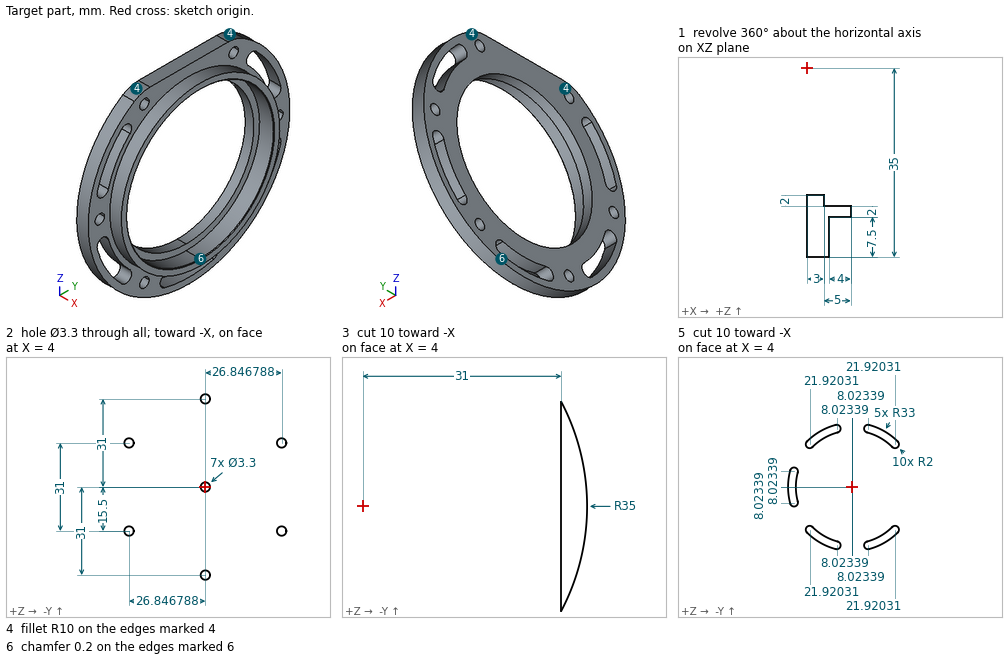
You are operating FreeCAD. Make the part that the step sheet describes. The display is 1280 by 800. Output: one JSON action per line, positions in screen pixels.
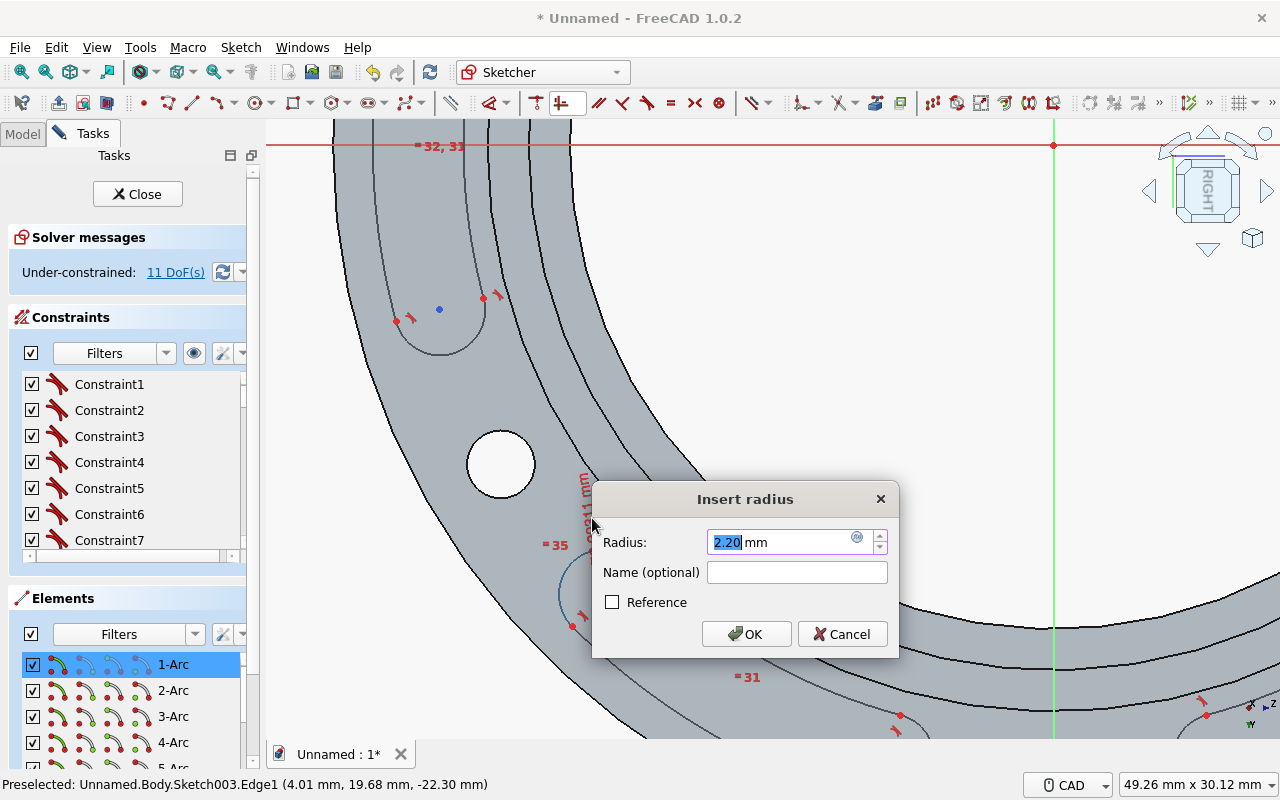
{"action": "type", "text": "2"}
{"action": "key", "text": "Return"}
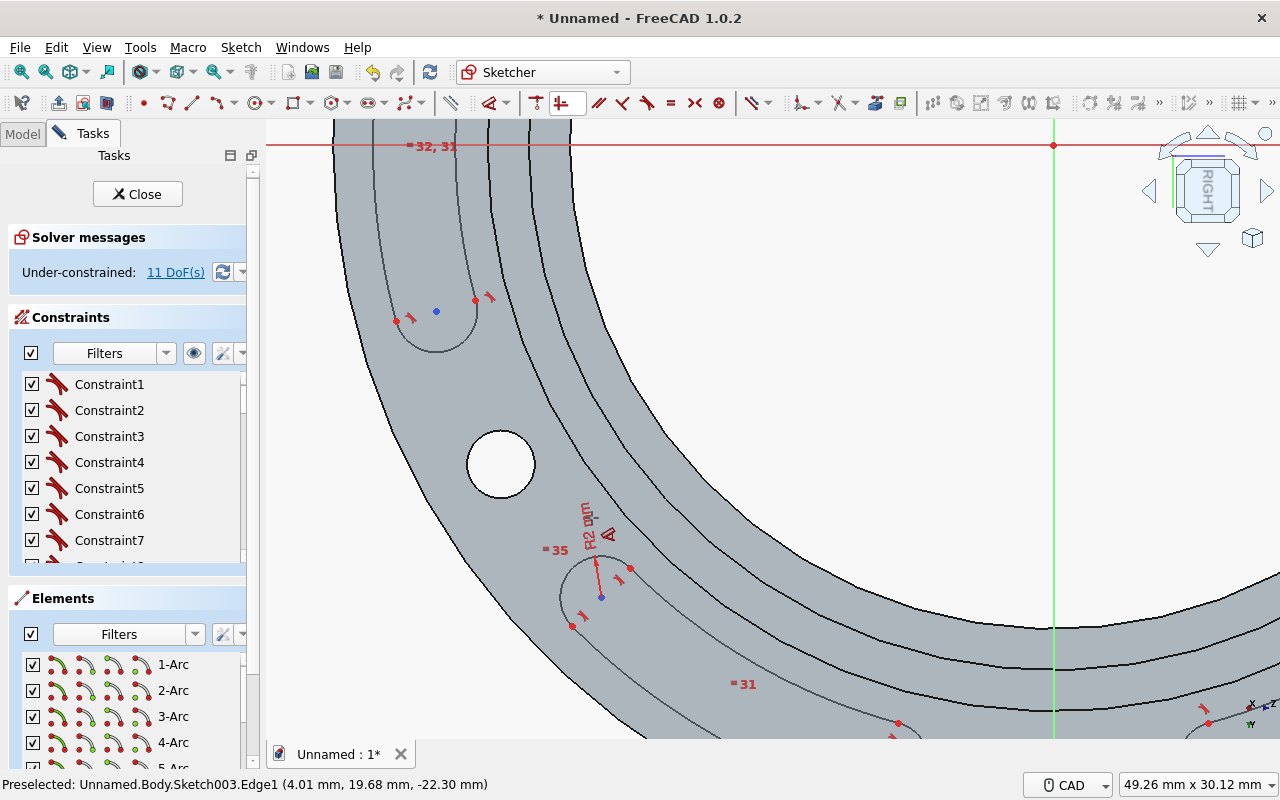
{"action": "left_click", "coordinate": [654, 696]}
{"action": "left_click", "coordinate": [410, 451]}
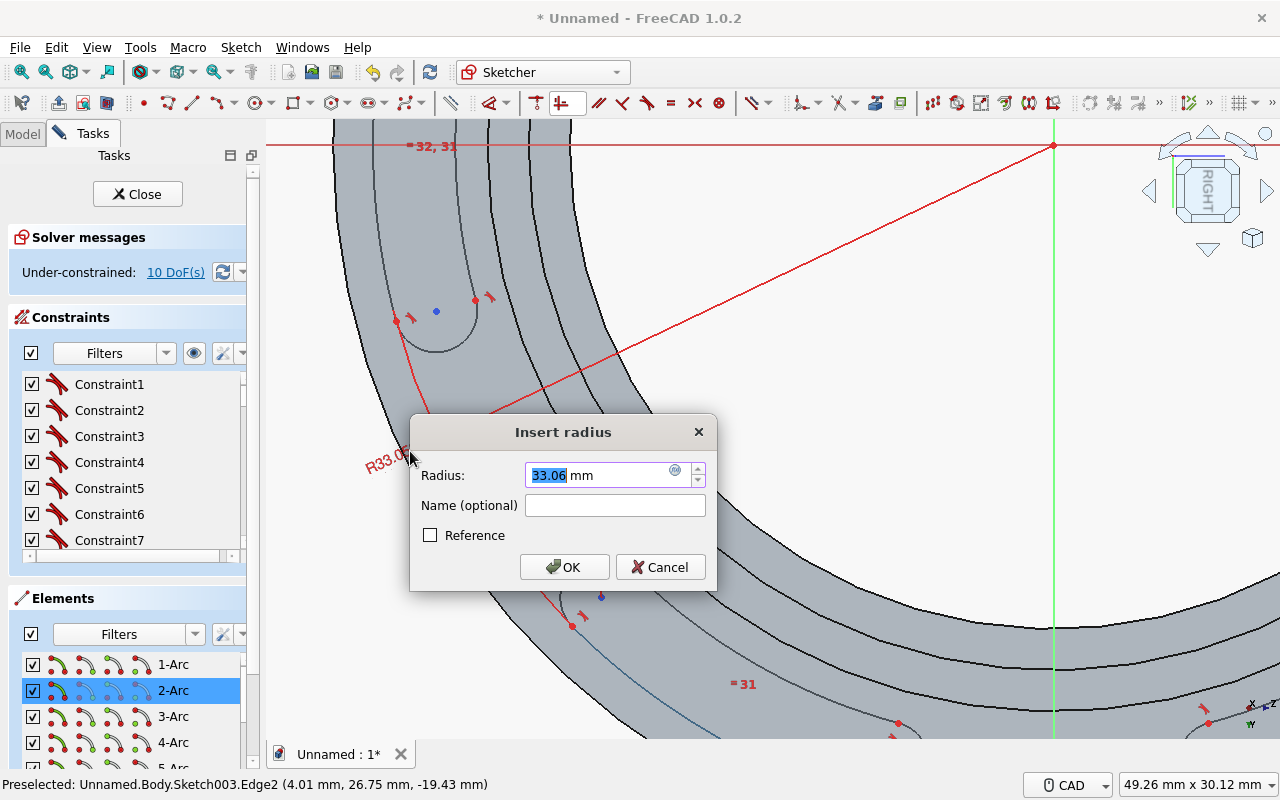
{"action": "type", "text": "33"}
{"action": "key", "text": "Return"}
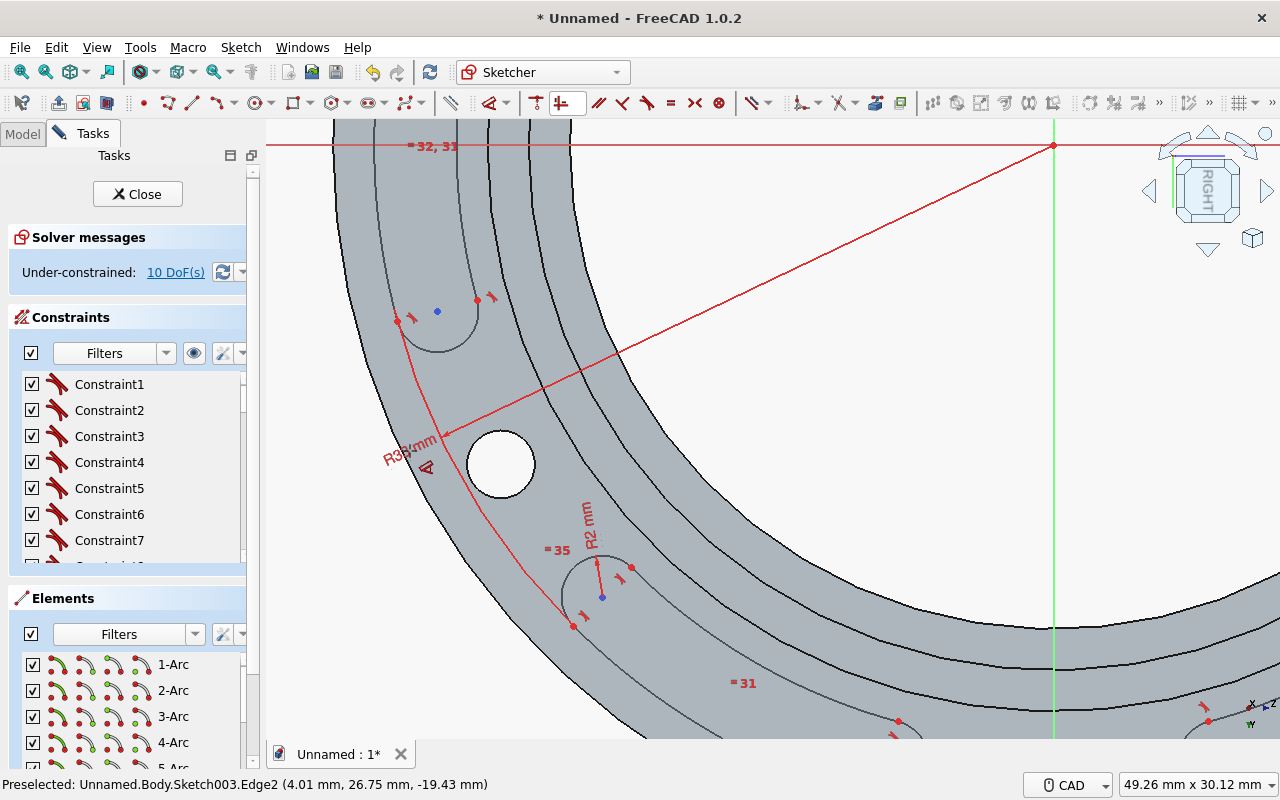
{"action": "scroll", "coordinate": [597, 551], "scroll_direction": "down", "scroll_amount": 6}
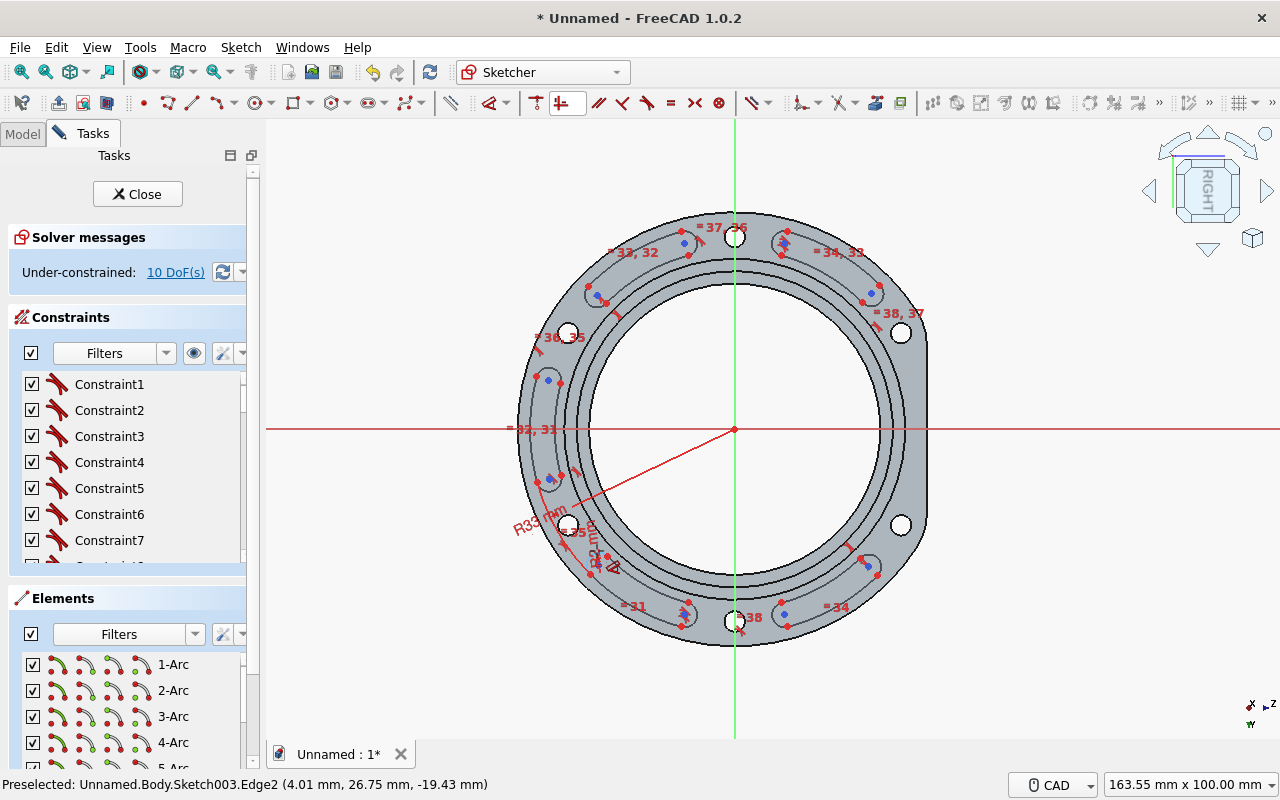
{"action": "left_click", "coordinate": [685, 615]}
{"action": "left_click", "coordinate": [710, 649]}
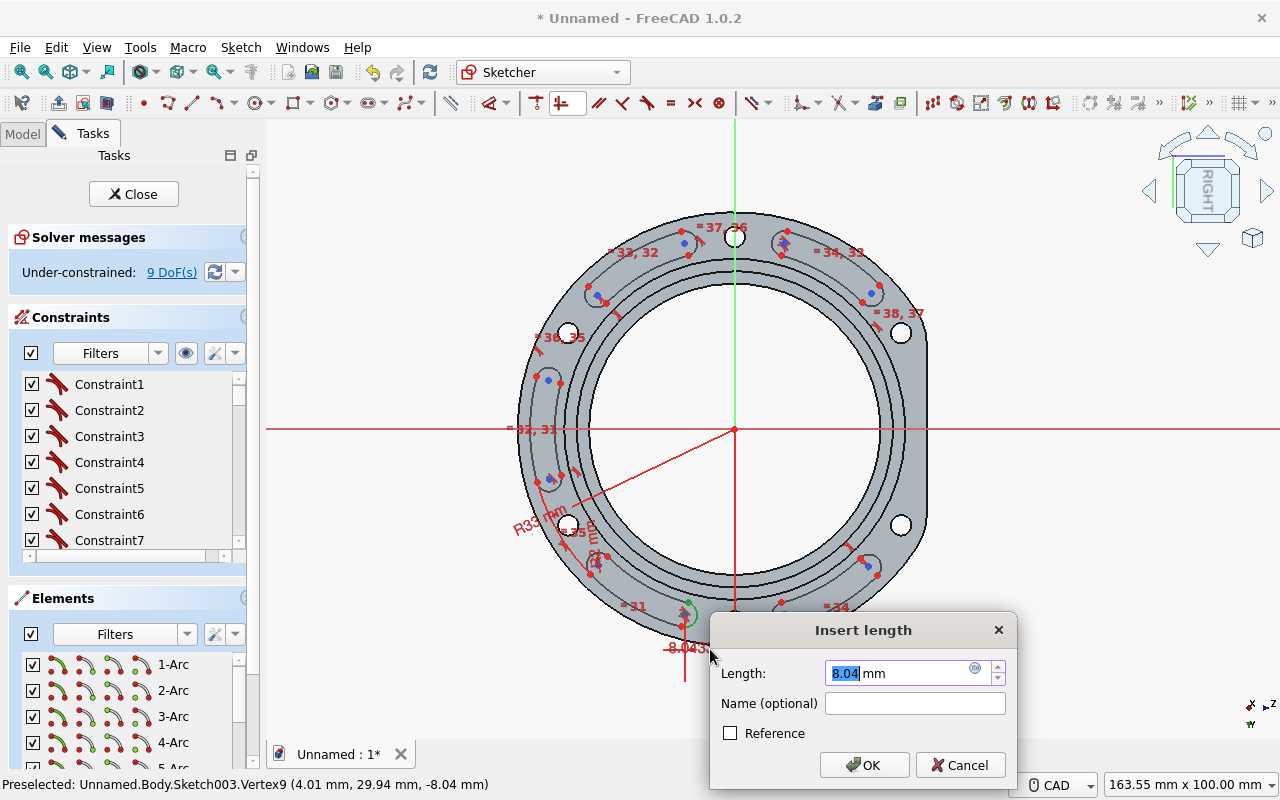
{"action": "type", "text": "8.02339"}
{"action": "key", "text": "Return"}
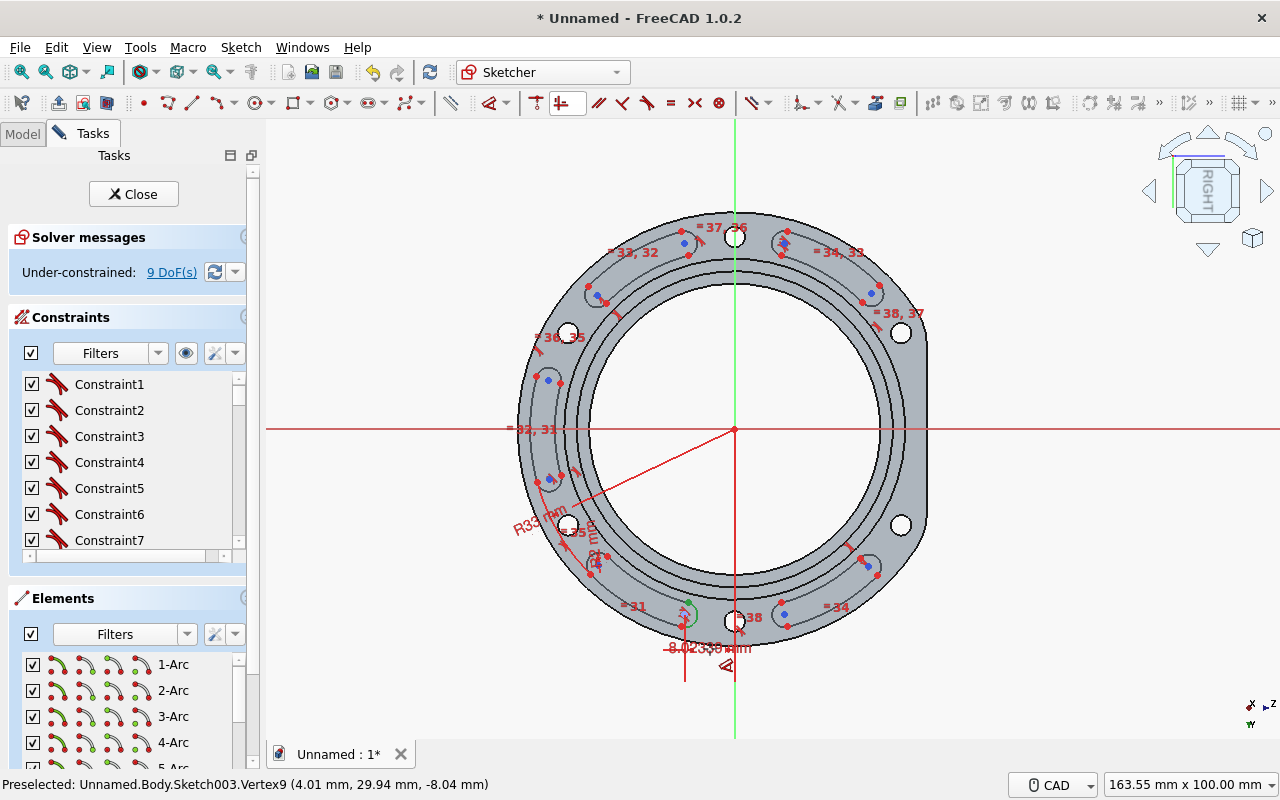
{"action": "left_click", "coordinate": [549, 380]}
{"action": "left_click", "coordinate": [515, 405]}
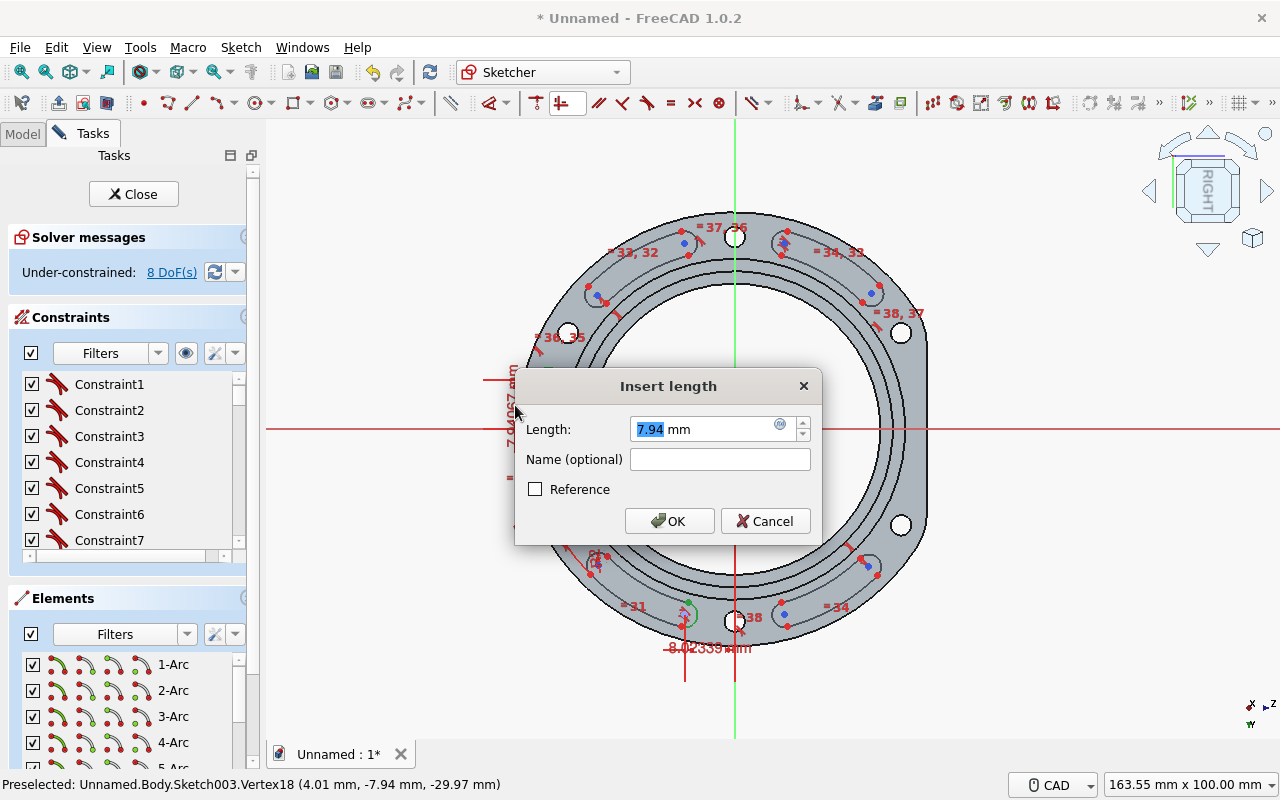
{"action": "type", "text": "8.02339"}
{"action": "key", "text": "Return"}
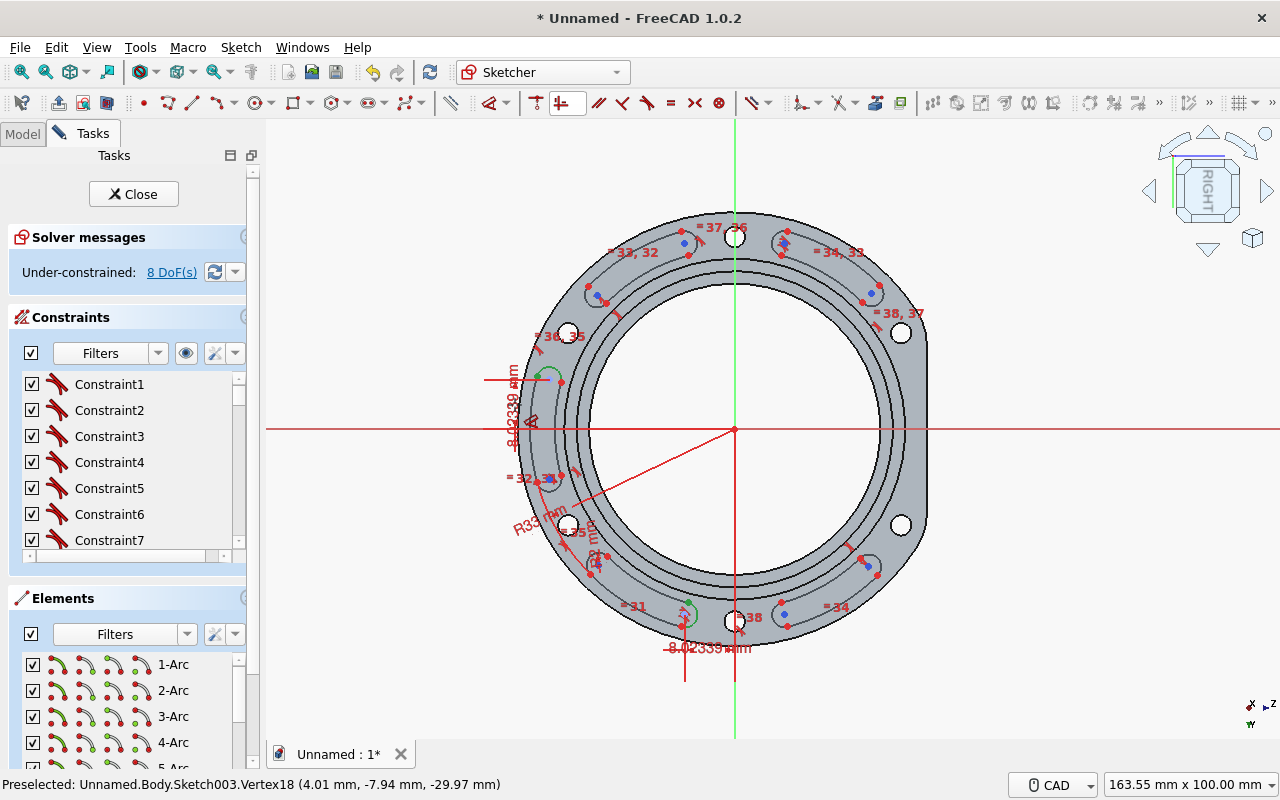
{"action": "left_click", "coordinate": [549, 479]}
{"action": "left_click", "coordinate": [515, 454]}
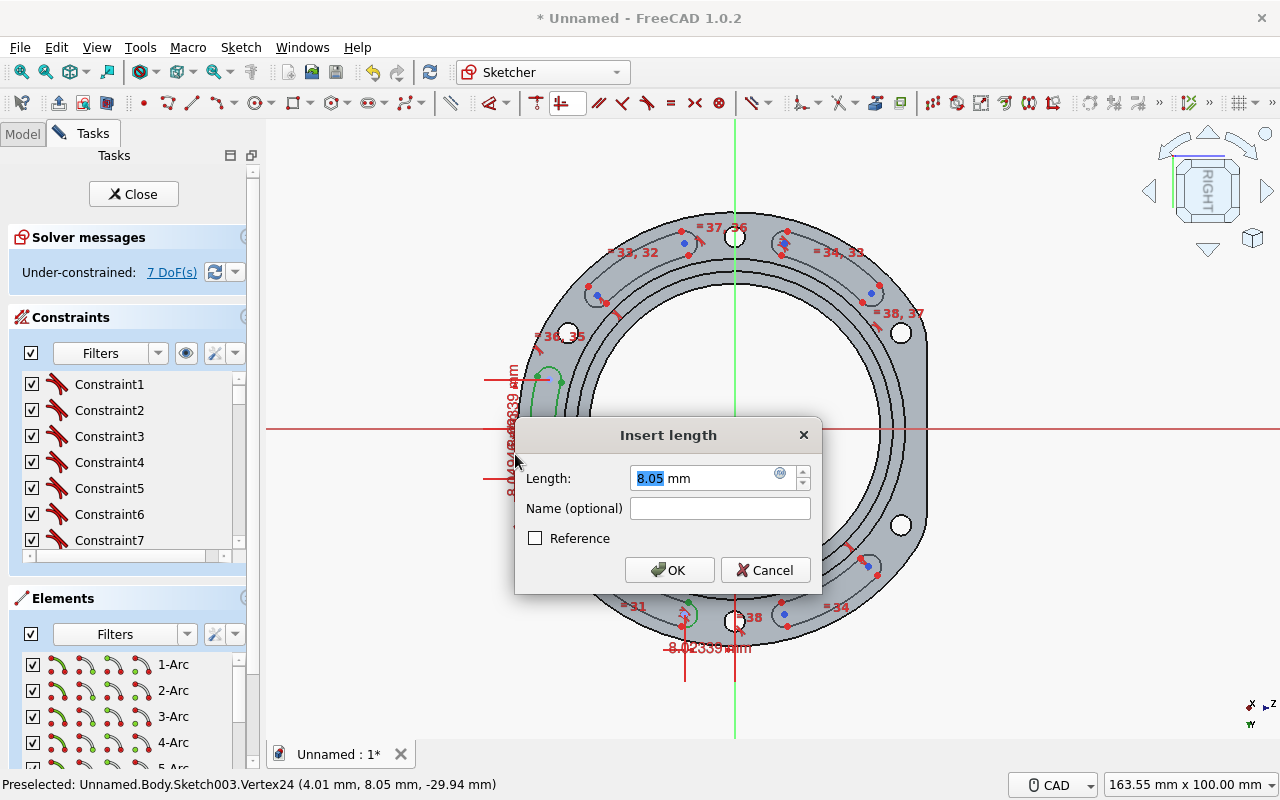
{"action": "type", "text": "8.02339"}
{"action": "key", "text": "Return"}